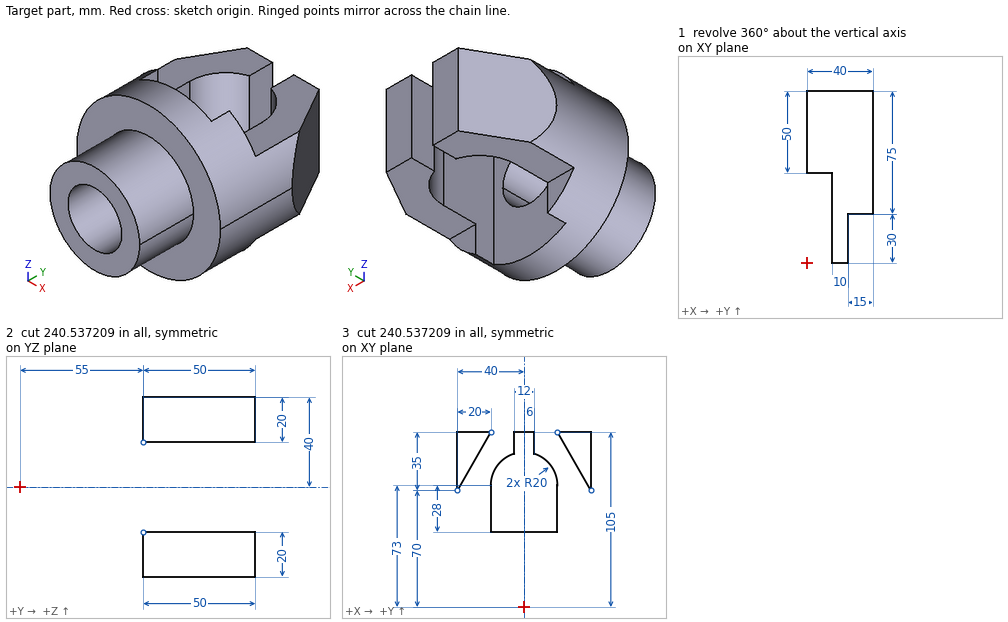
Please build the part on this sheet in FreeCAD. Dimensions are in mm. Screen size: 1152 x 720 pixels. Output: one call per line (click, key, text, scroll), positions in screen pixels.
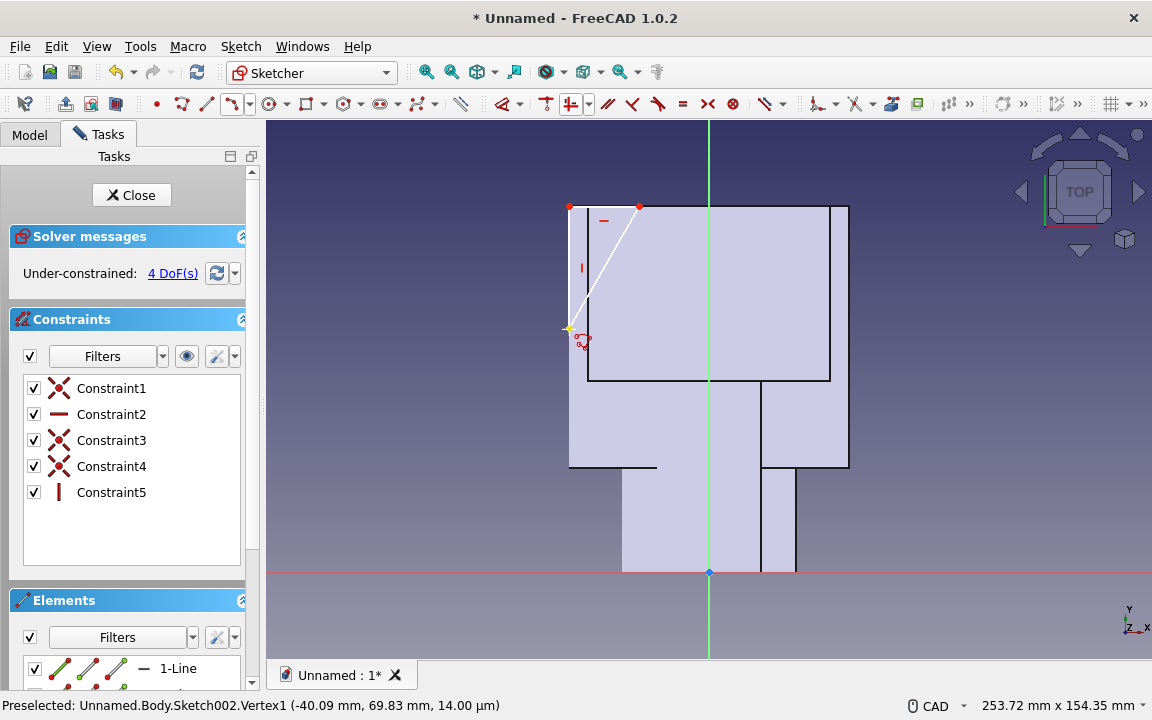
click(849, 328)
click(849, 206)
click(779, 206)
click(849, 329)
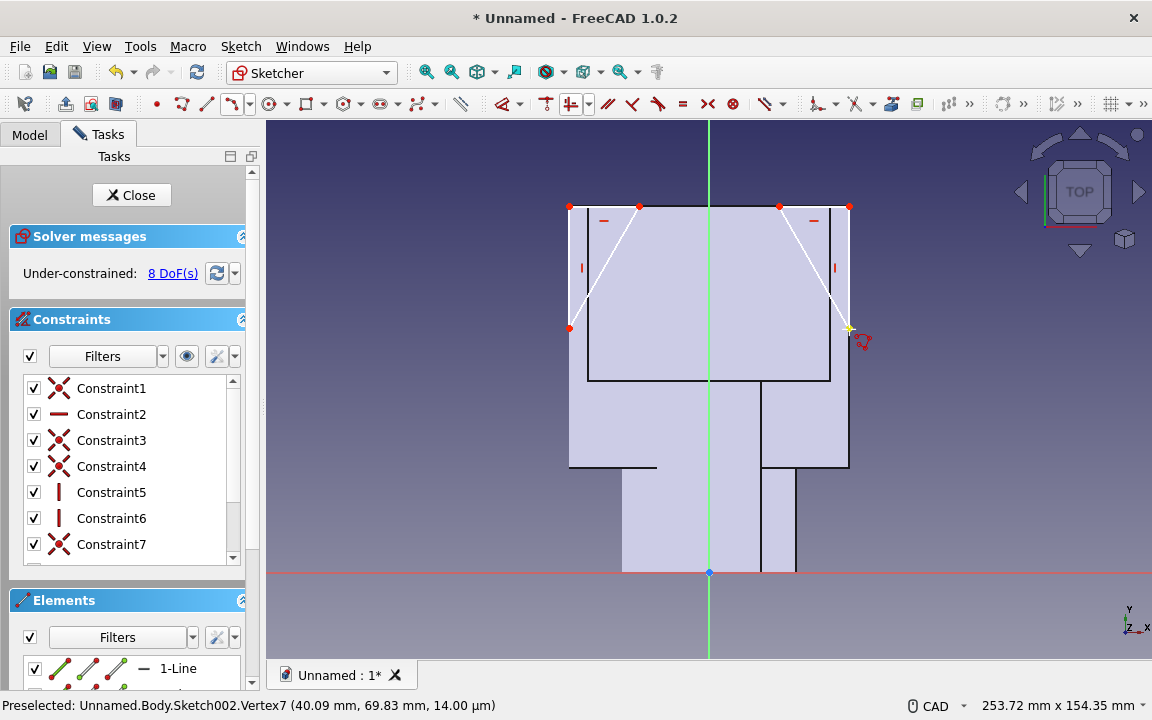
click(730, 251)
click(730, 206)
click(688, 206)
click(688, 251)
right_click(688, 251)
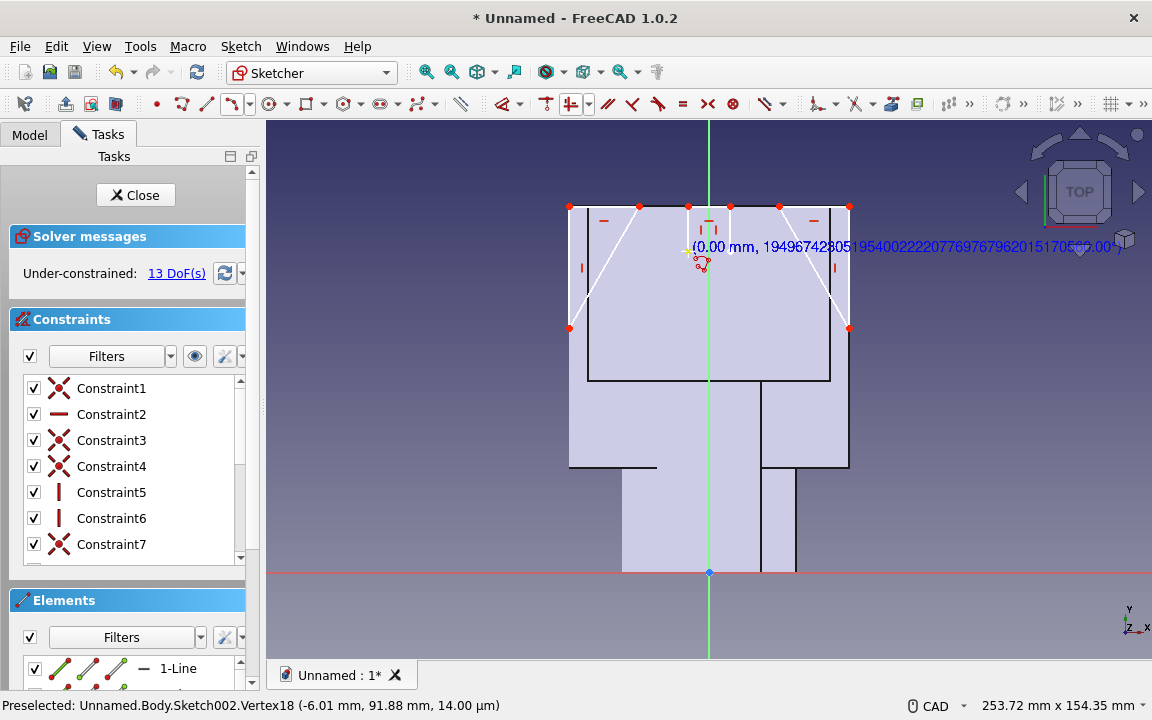
click(639, 318)
click(639, 416)
click(779, 416)
click(779, 318)
right_click(779, 318)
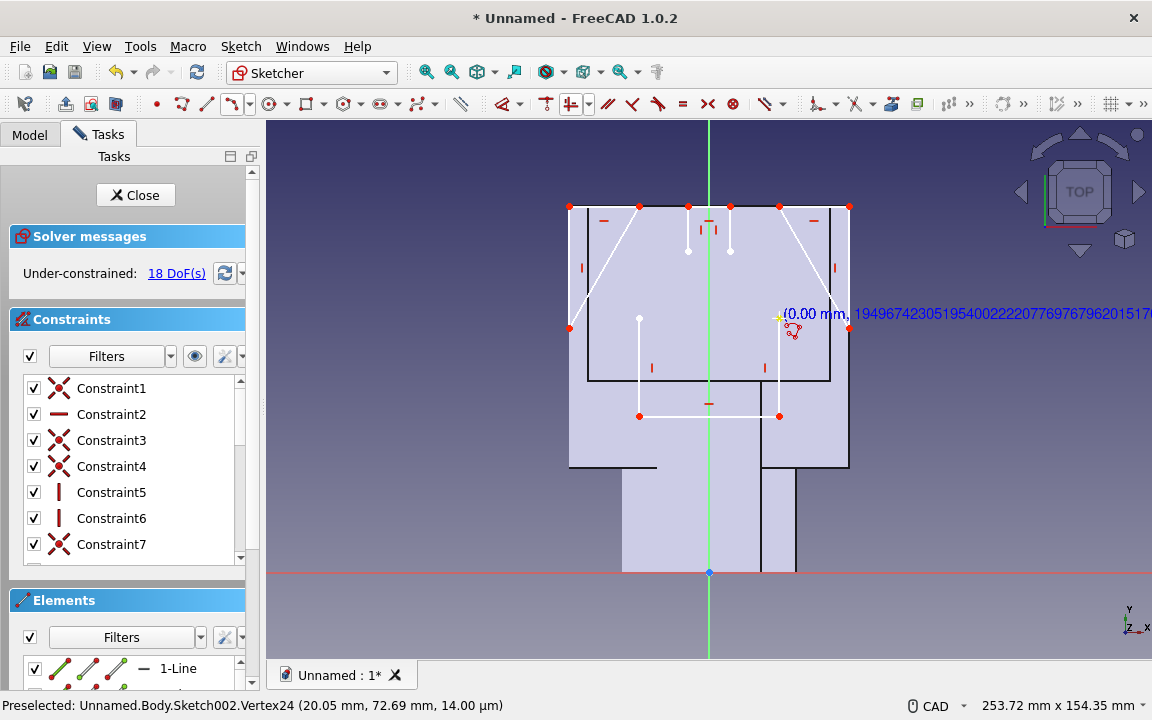
click(232, 104)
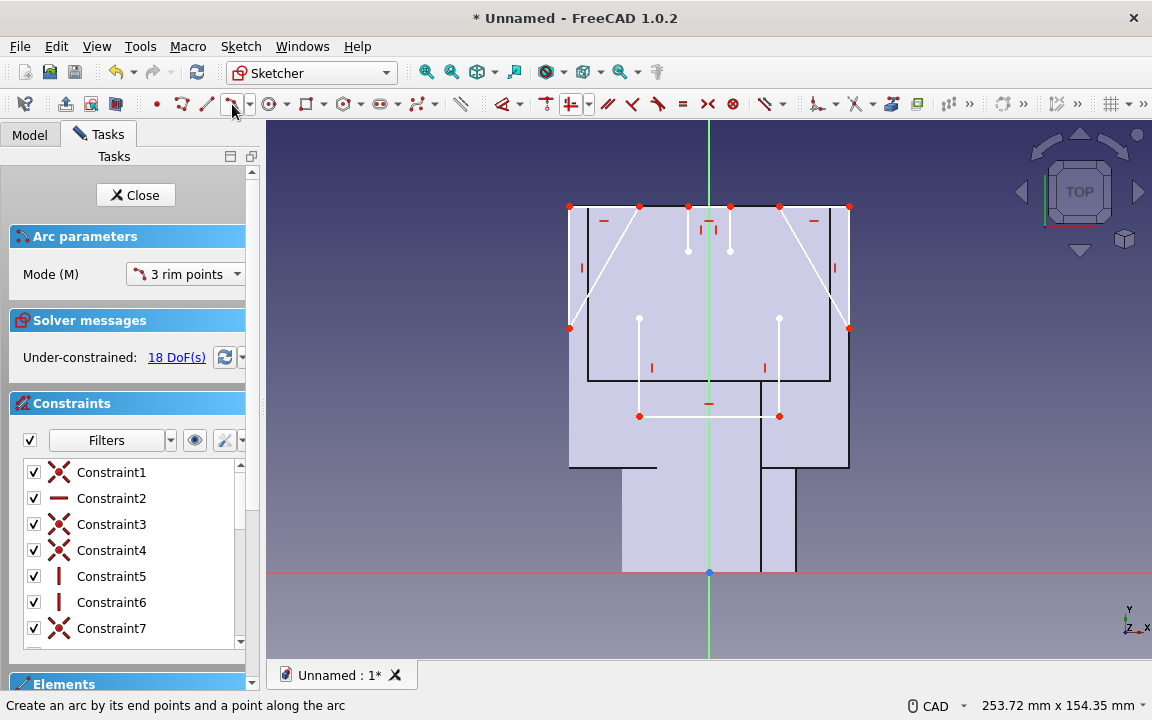
click(688, 252)
click(639, 319)
click(653, 277)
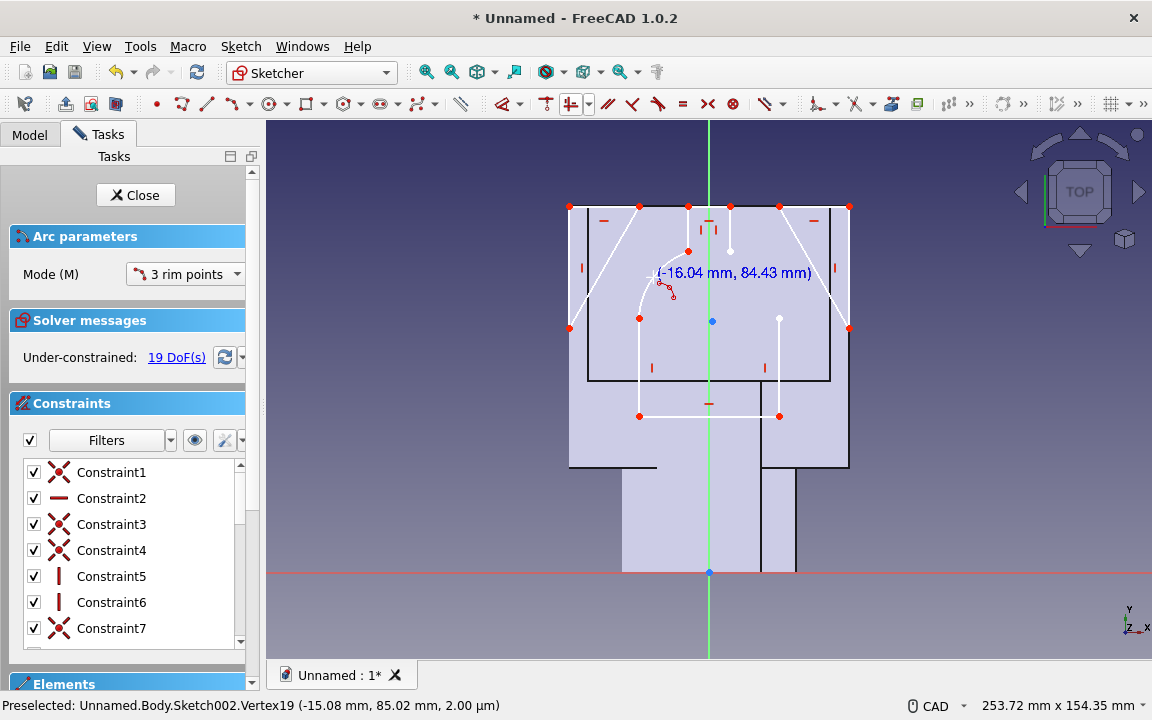
click(779, 319)
click(730, 252)
click(765, 277)
key(Escape)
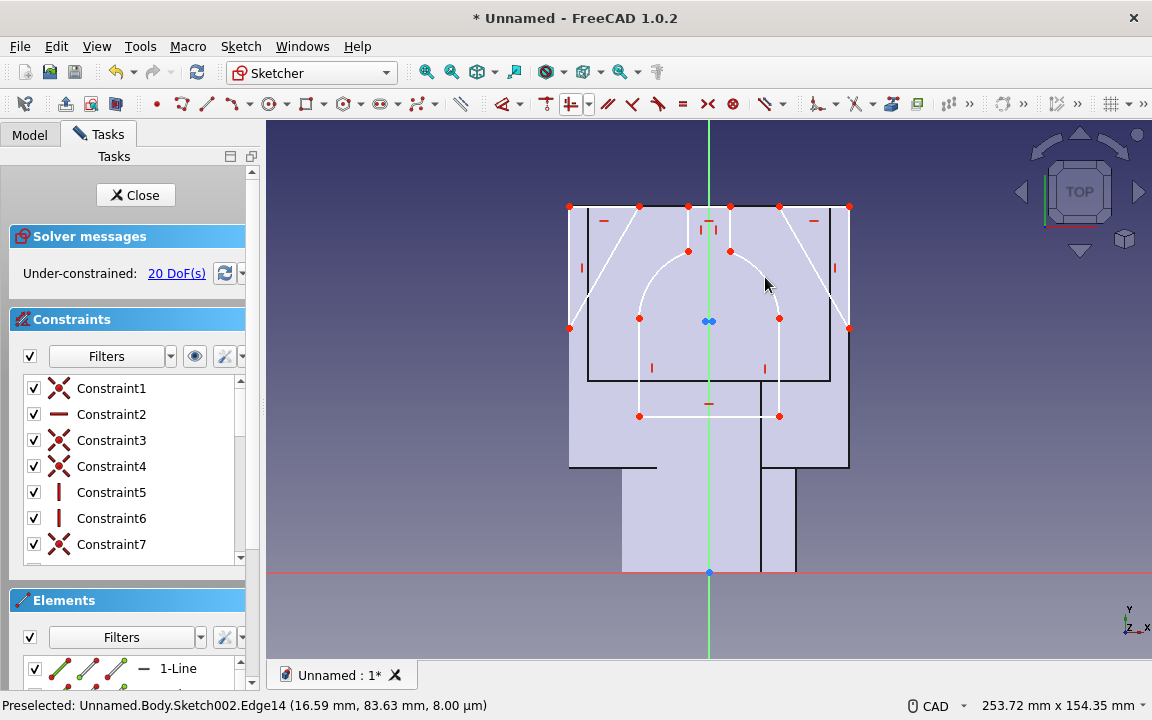
click(639, 348)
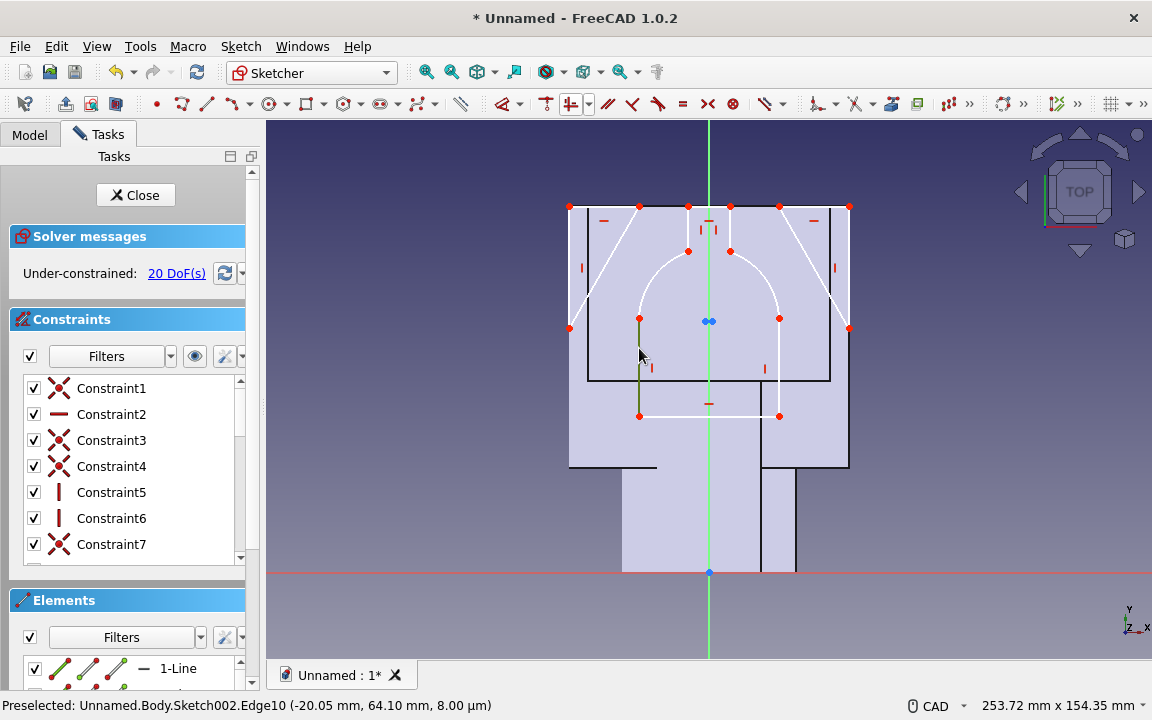
click(665, 265)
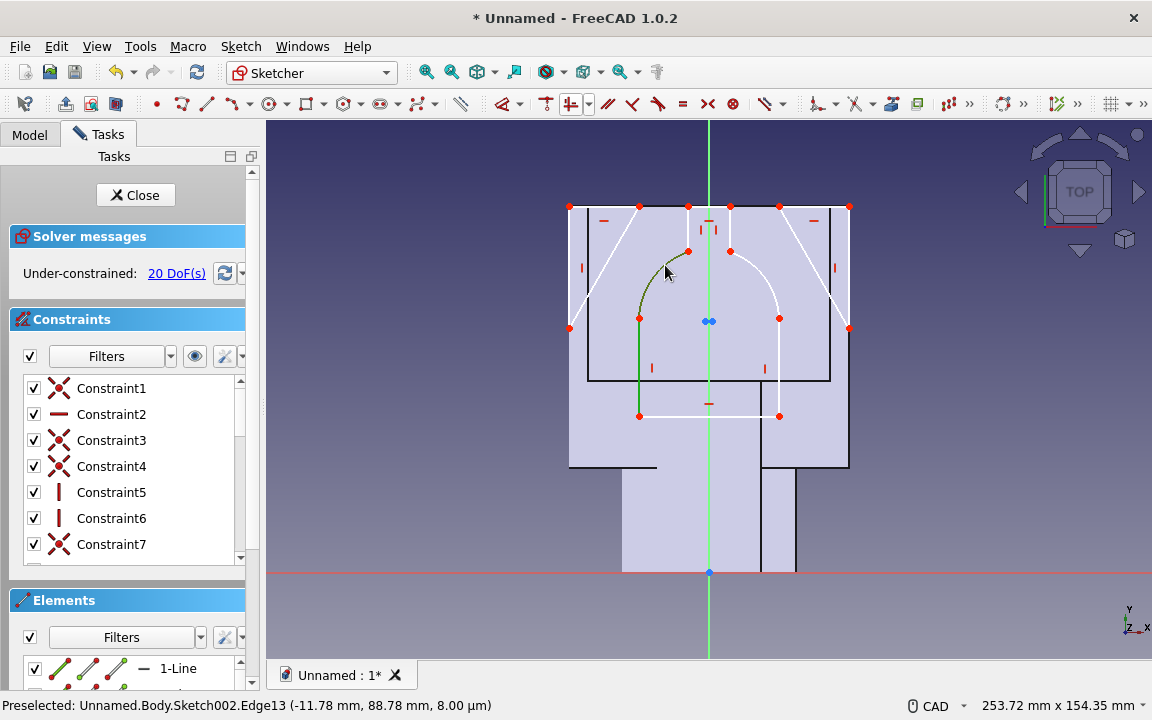
click(658, 104)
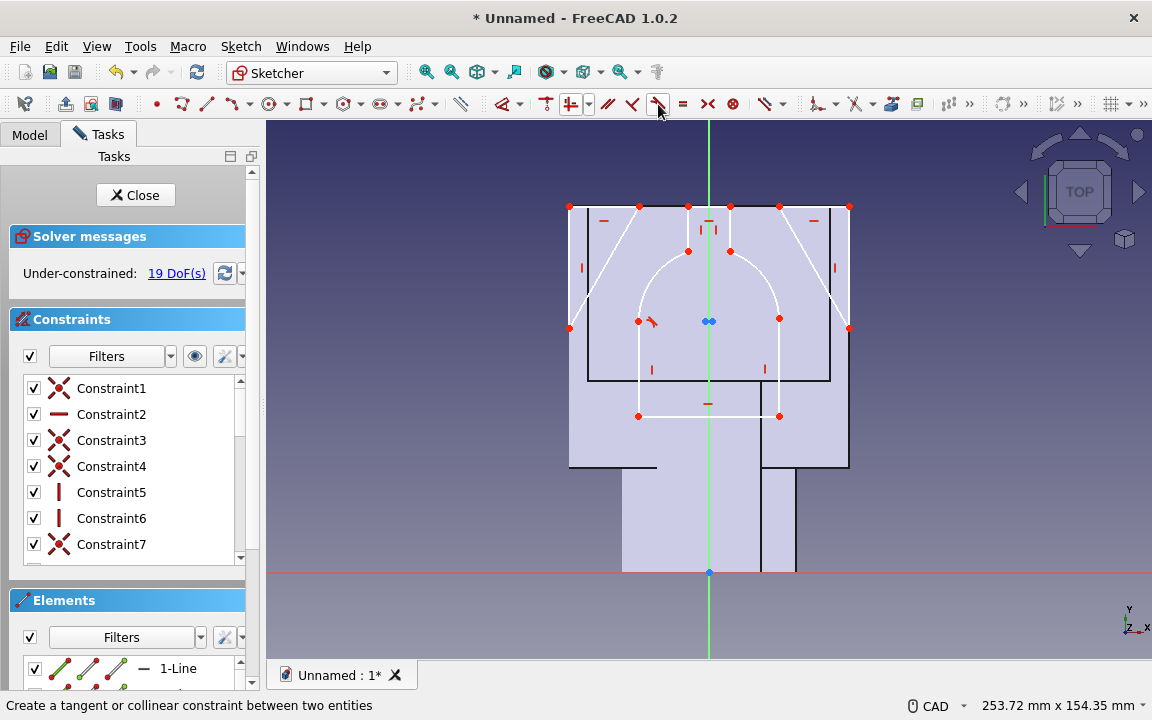
click(779, 388)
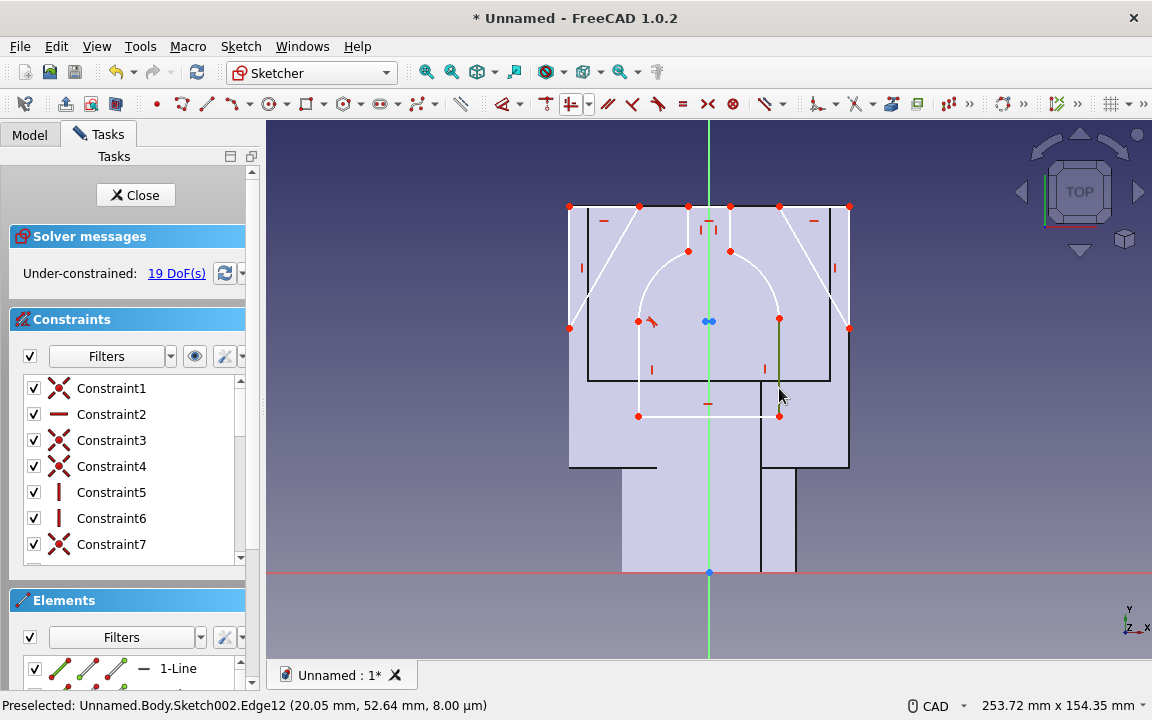
click(774, 293)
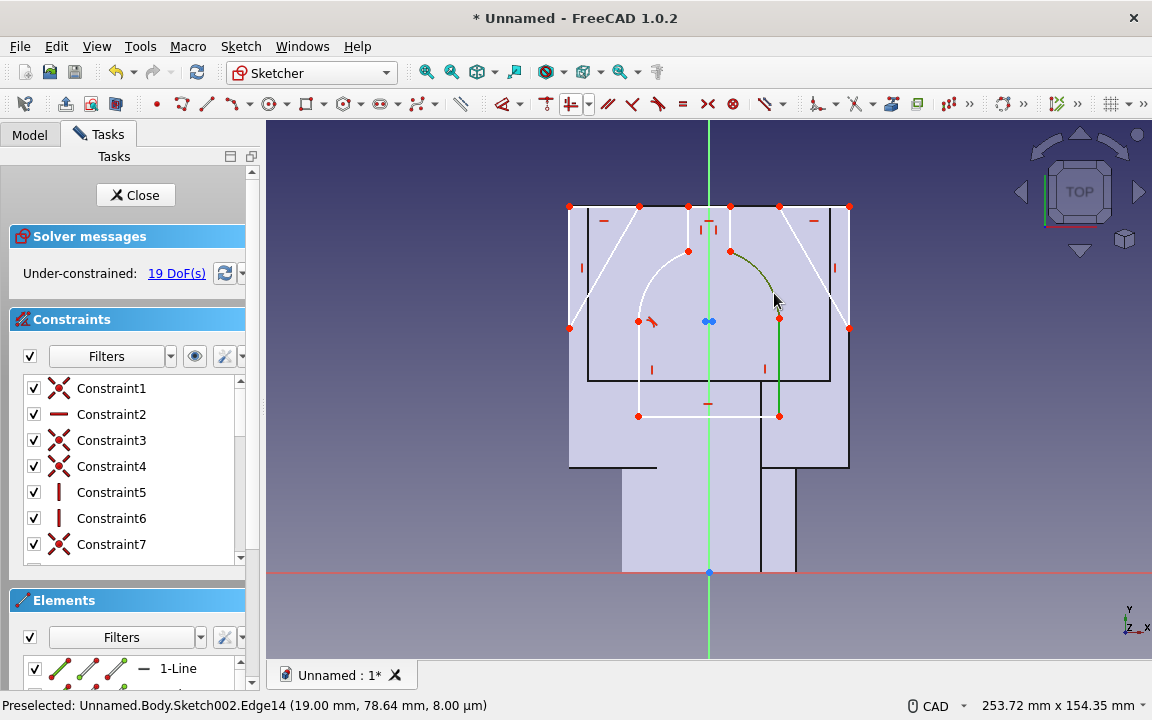
click(658, 104)